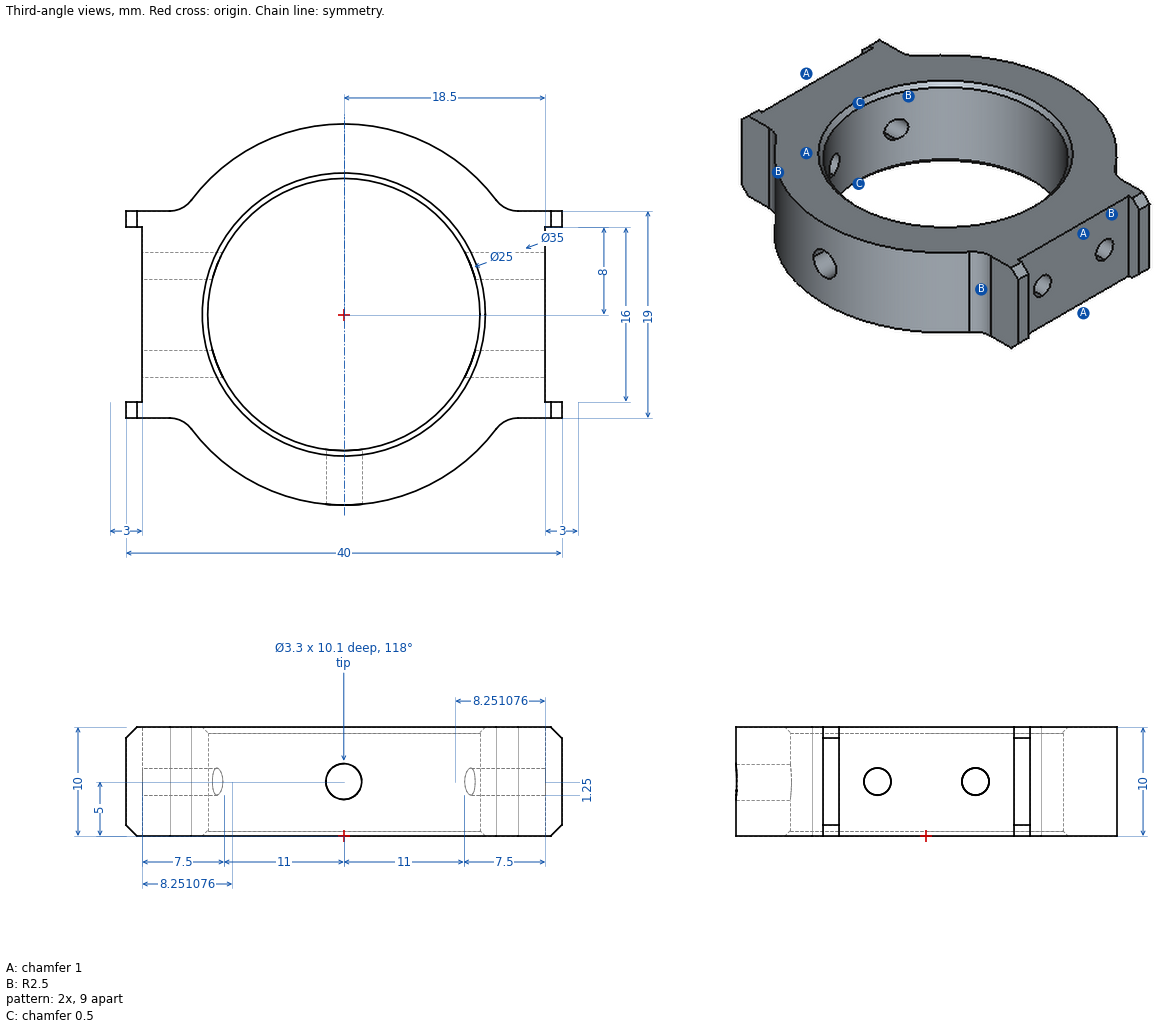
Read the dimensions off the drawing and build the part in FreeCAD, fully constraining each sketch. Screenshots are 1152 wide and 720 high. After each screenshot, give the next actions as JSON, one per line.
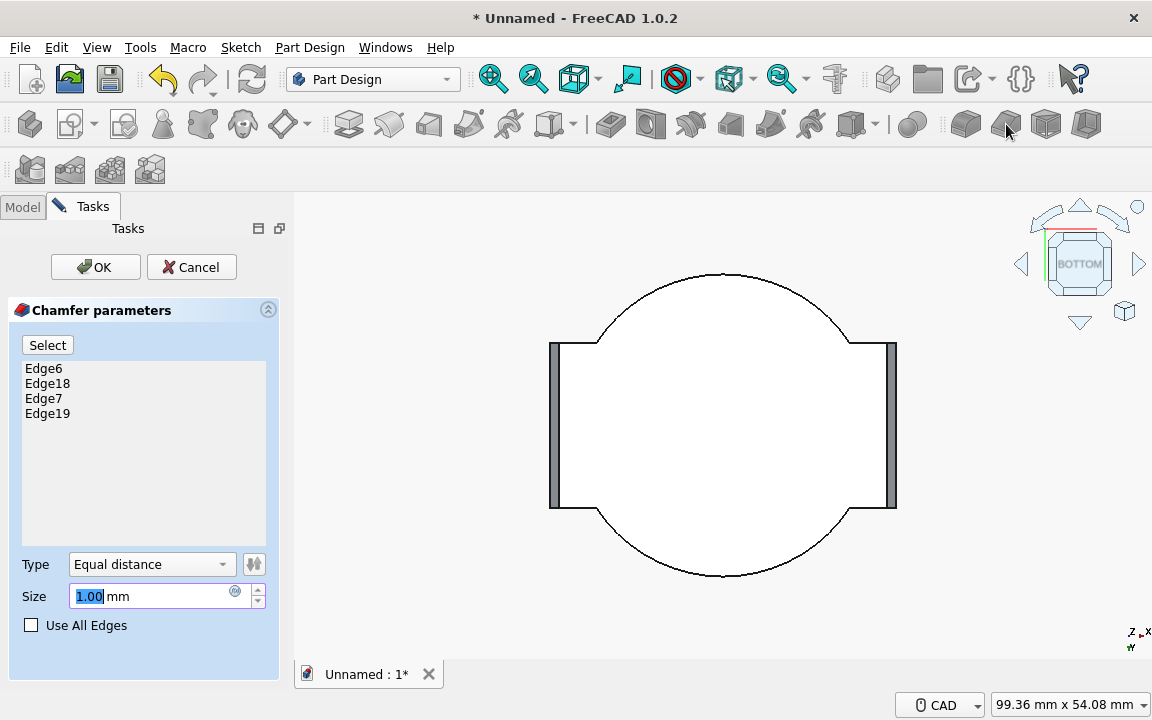
{"action": "type", "text": "1"}
{"action": "key", "text": "Tab"}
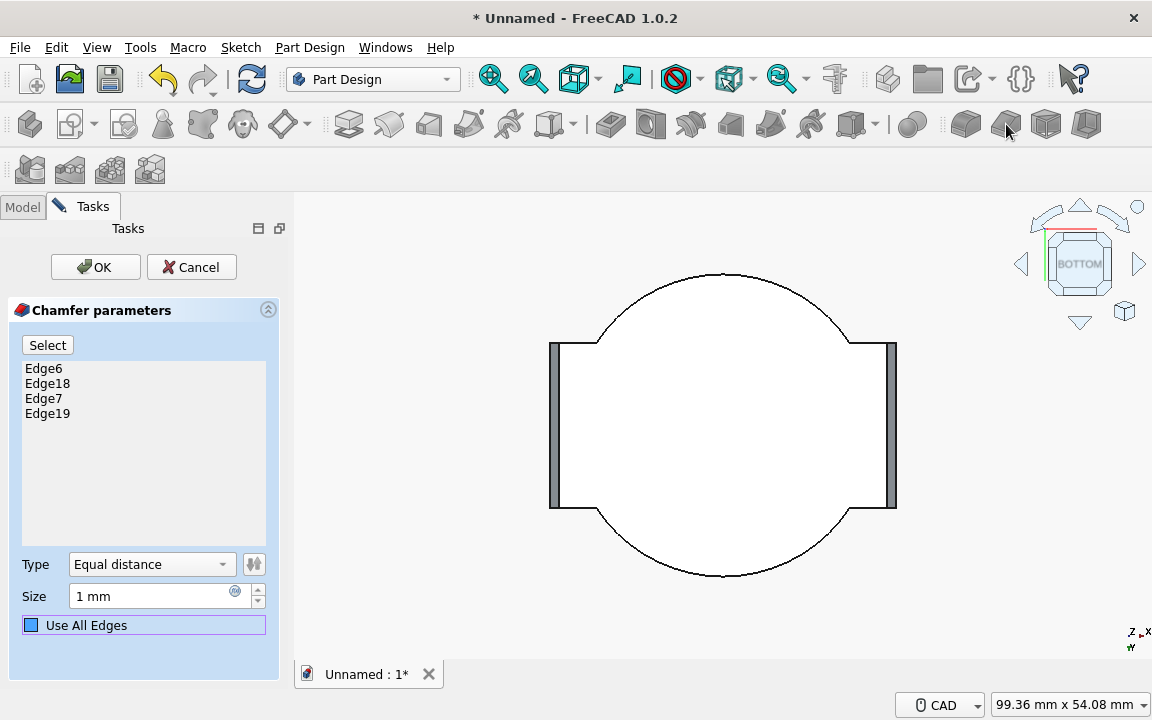
{"action": "left_click", "coordinate": [96, 267]}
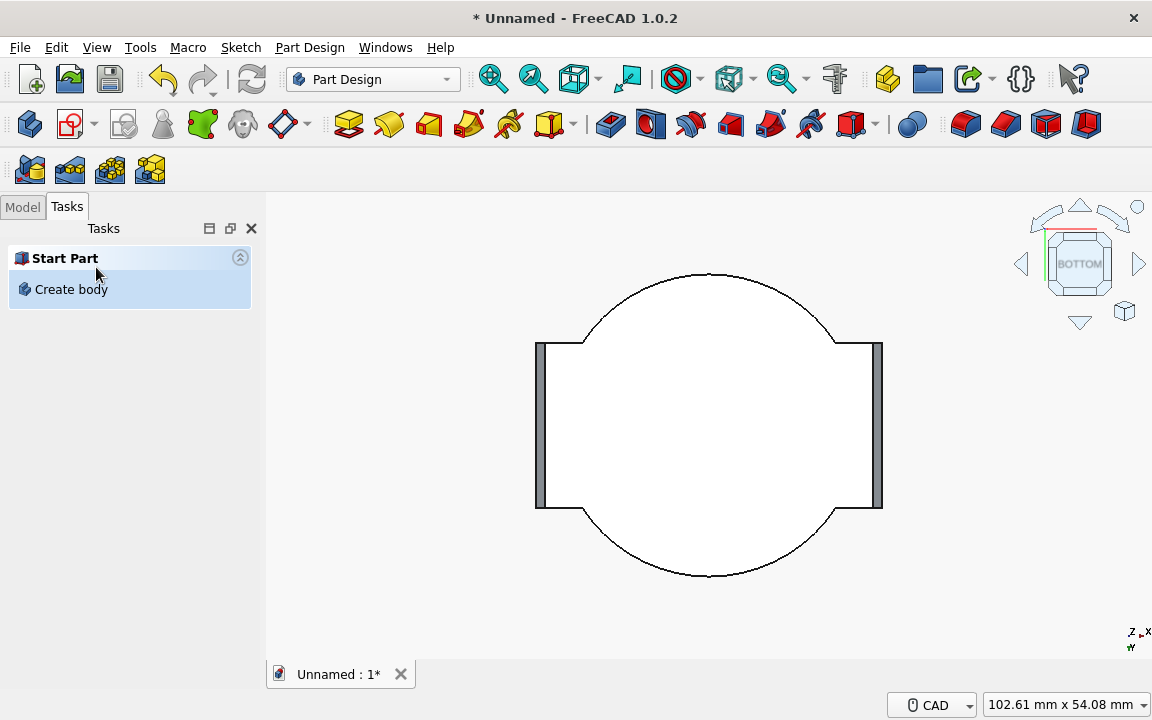
{"action": "key", "text": "0"}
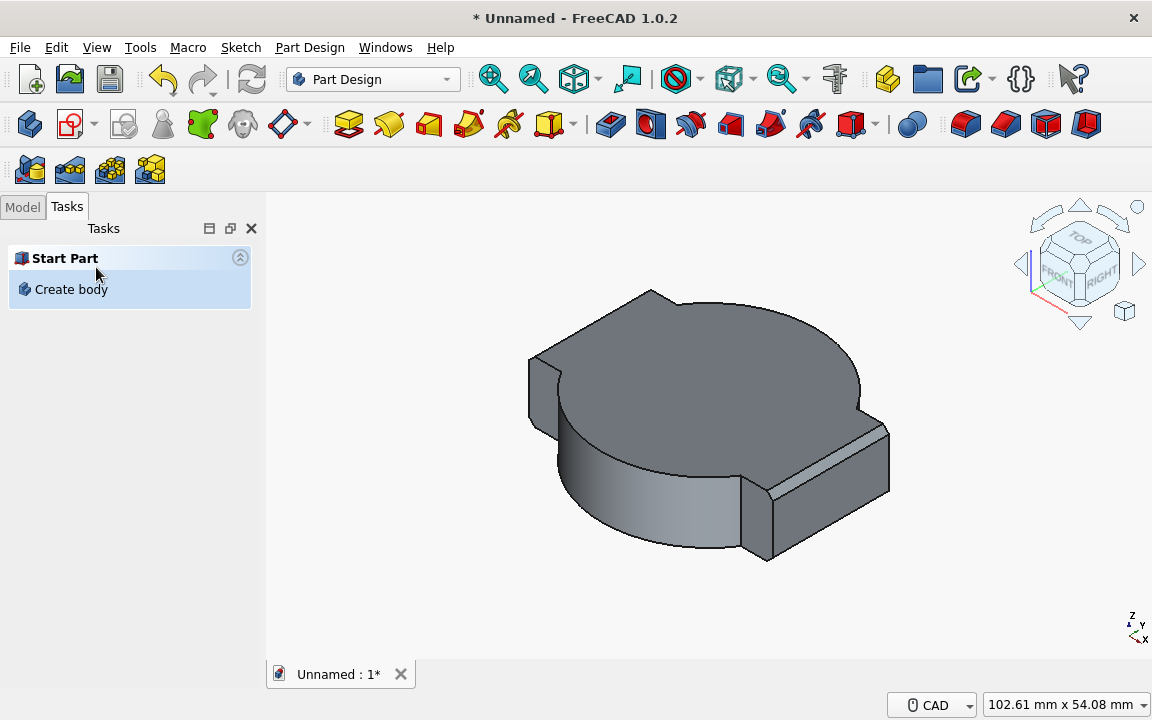
{"action": "left_click", "coordinate": [709, 389]}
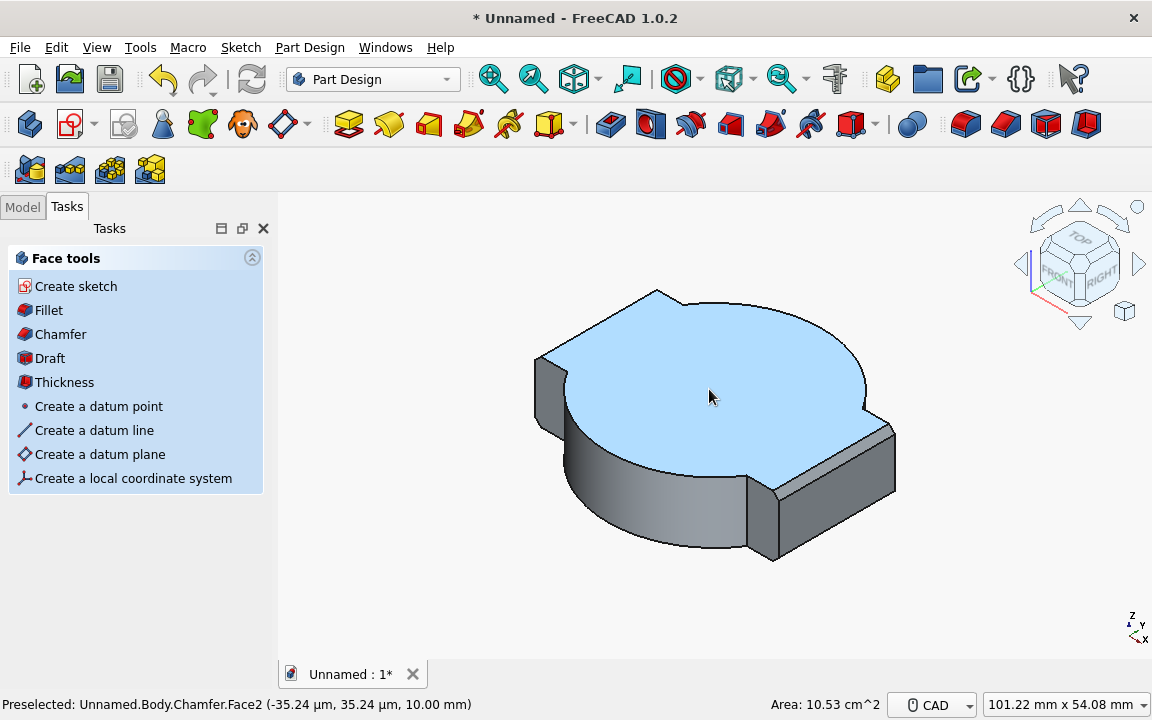
{"action": "left_click", "coordinate": [70, 124]}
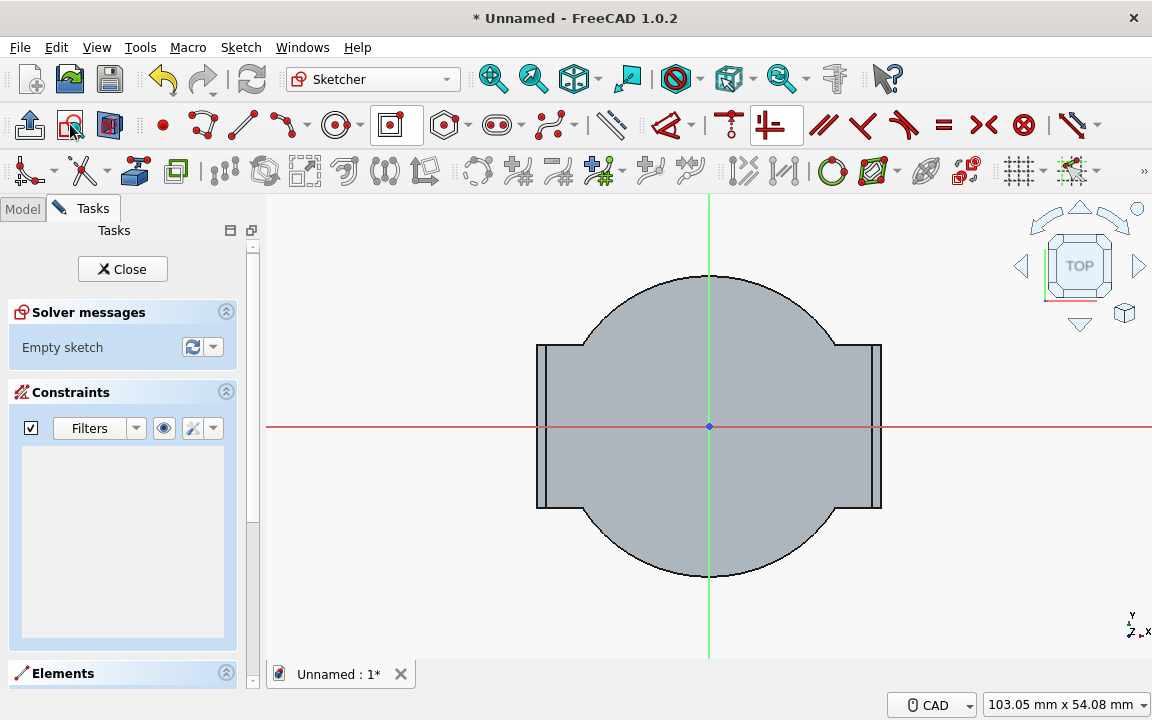
{"action": "left_click", "coordinate": [336, 126]}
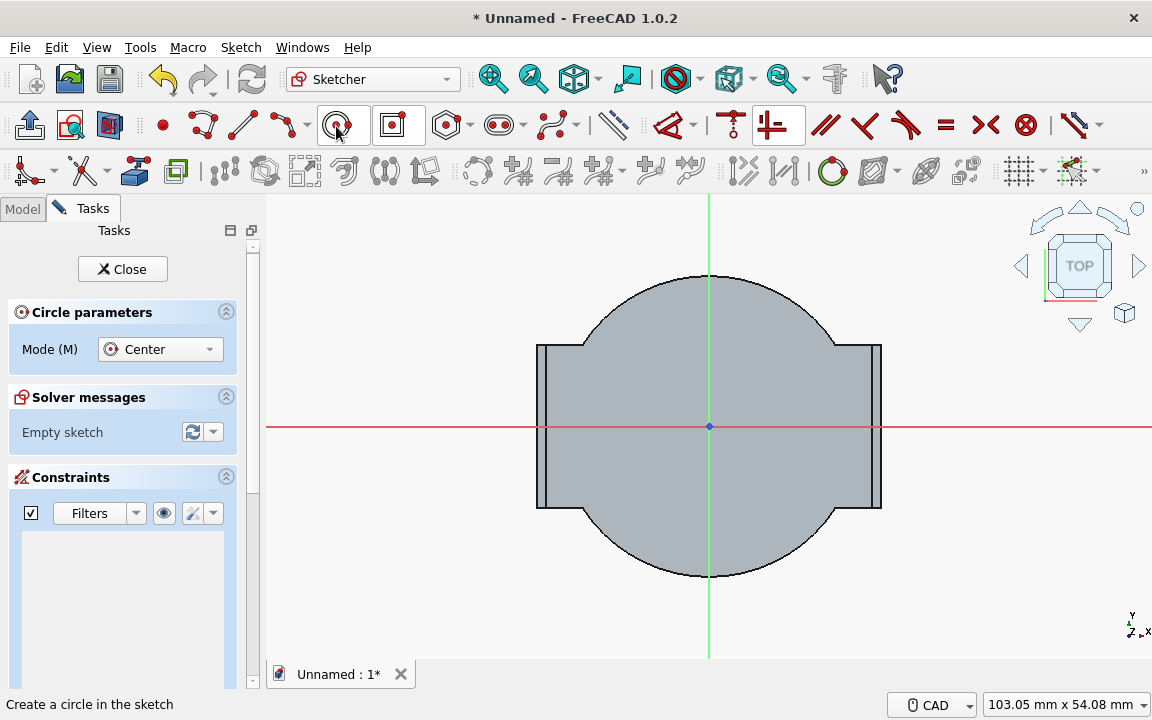
{"action": "left_click", "coordinate": [709, 426]}
{"action": "mouse_move", "coordinate": [785, 351]}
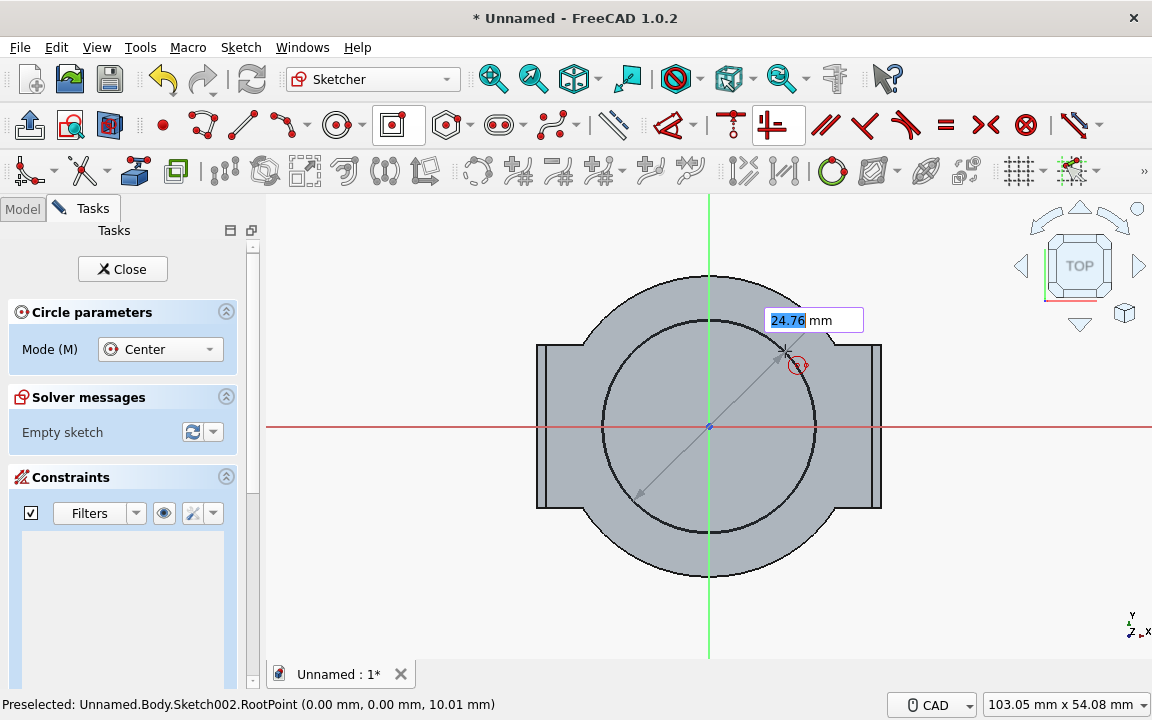
{"action": "type", "text": "25"}
{"action": "key", "text": "Return"}
{"action": "key", "text": "Escape"}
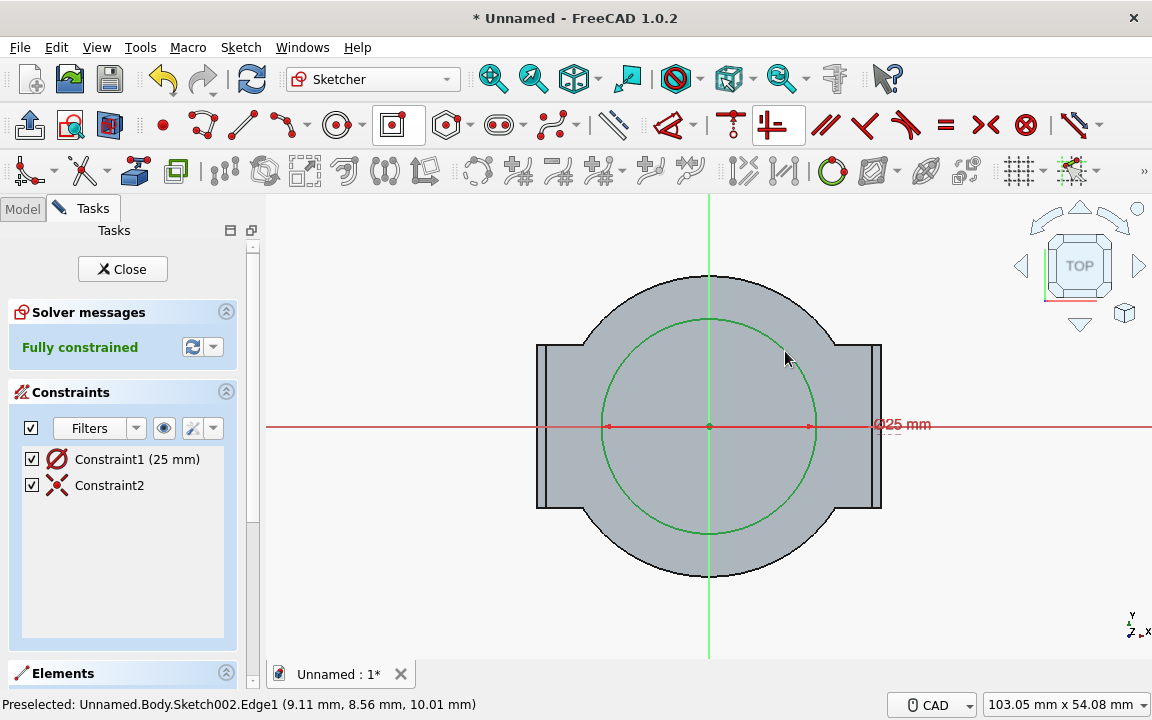
{"action": "left_click", "coordinate": [123, 269]}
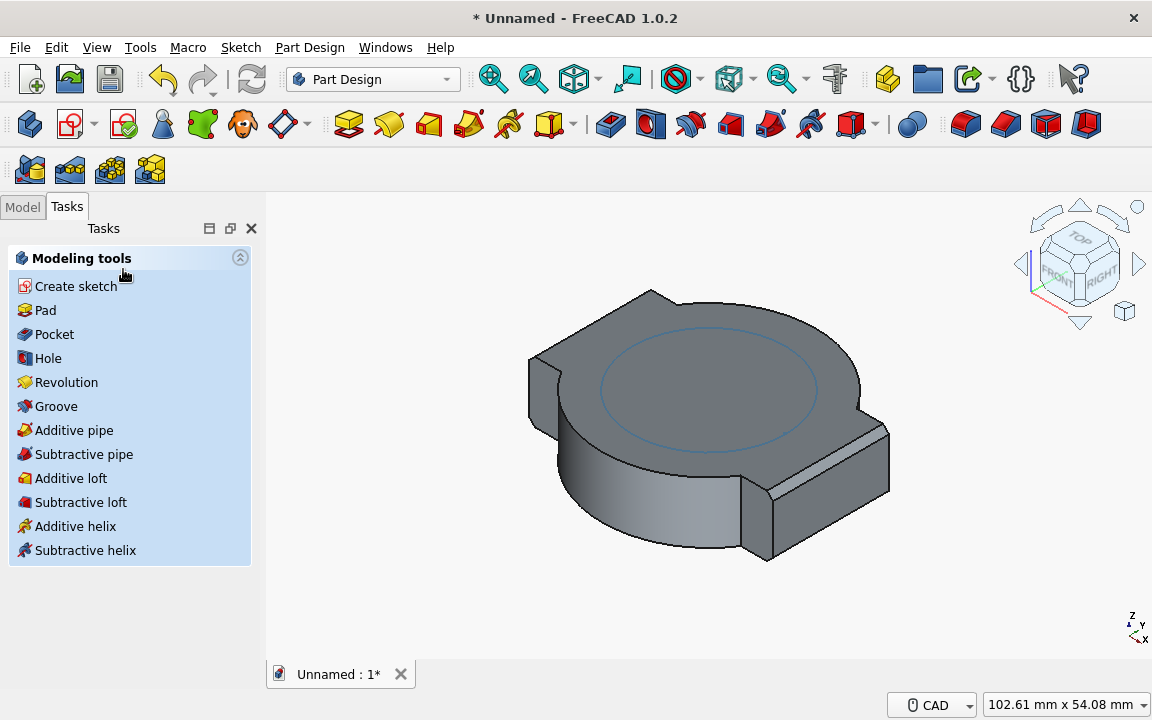
{"action": "left_click", "coordinate": [612, 124]}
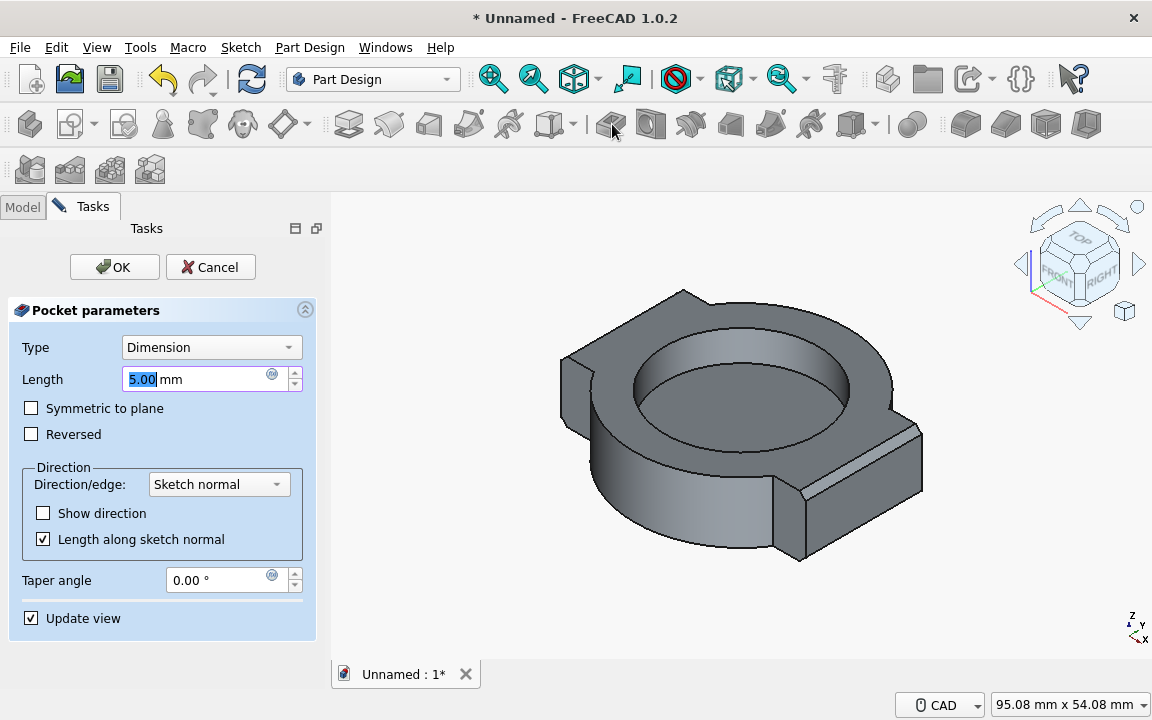
{"action": "left_click", "coordinate": [212, 348]}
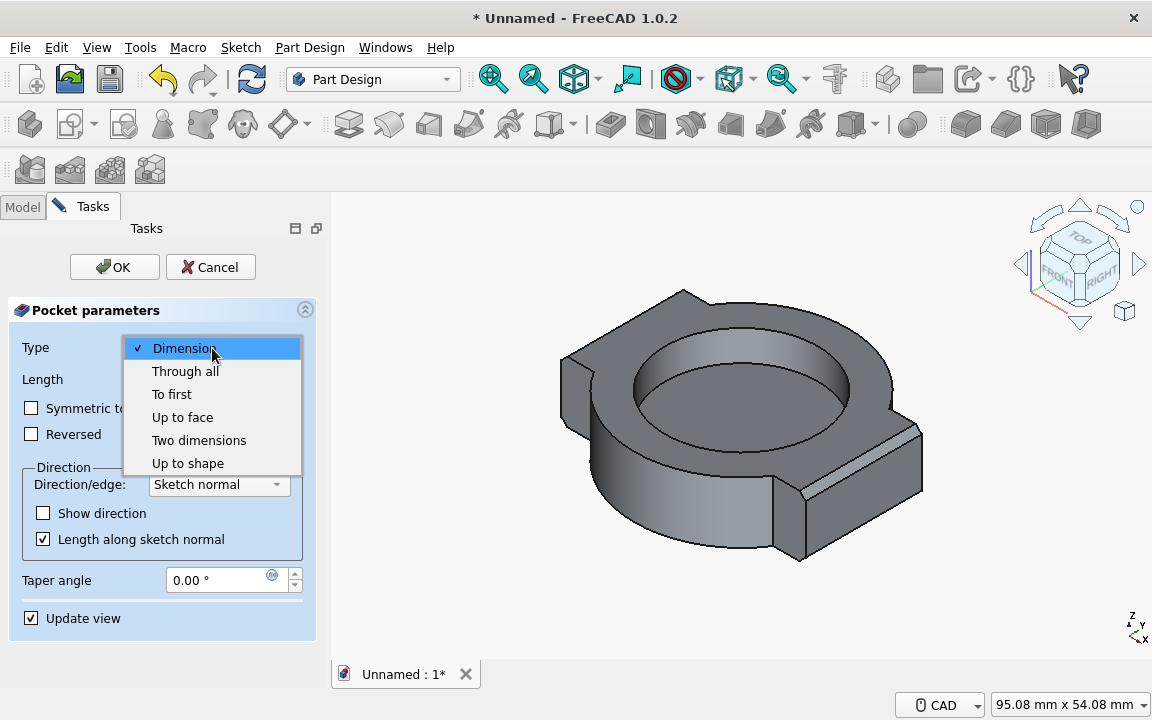
{"action": "left_click", "coordinate": [212, 372]}